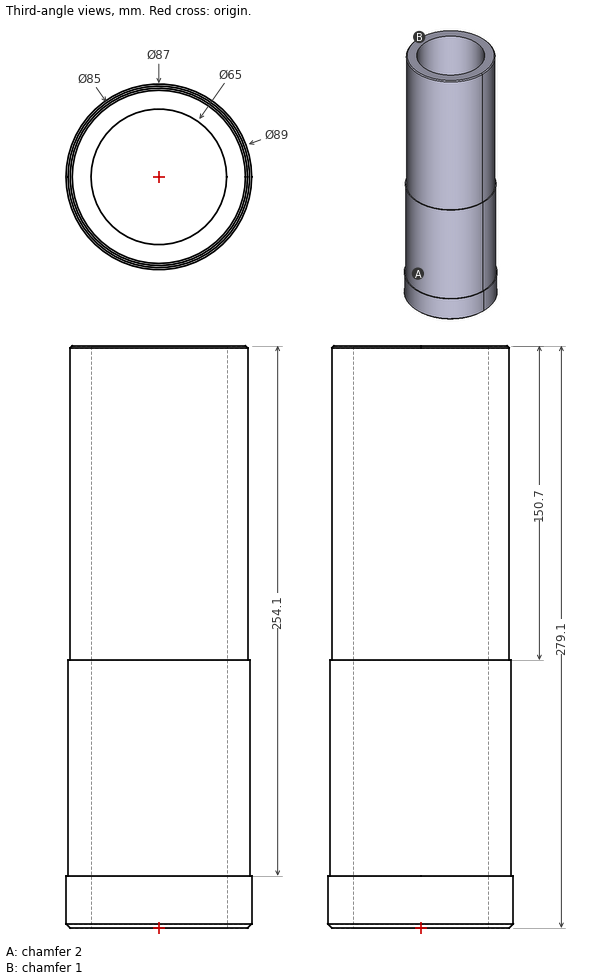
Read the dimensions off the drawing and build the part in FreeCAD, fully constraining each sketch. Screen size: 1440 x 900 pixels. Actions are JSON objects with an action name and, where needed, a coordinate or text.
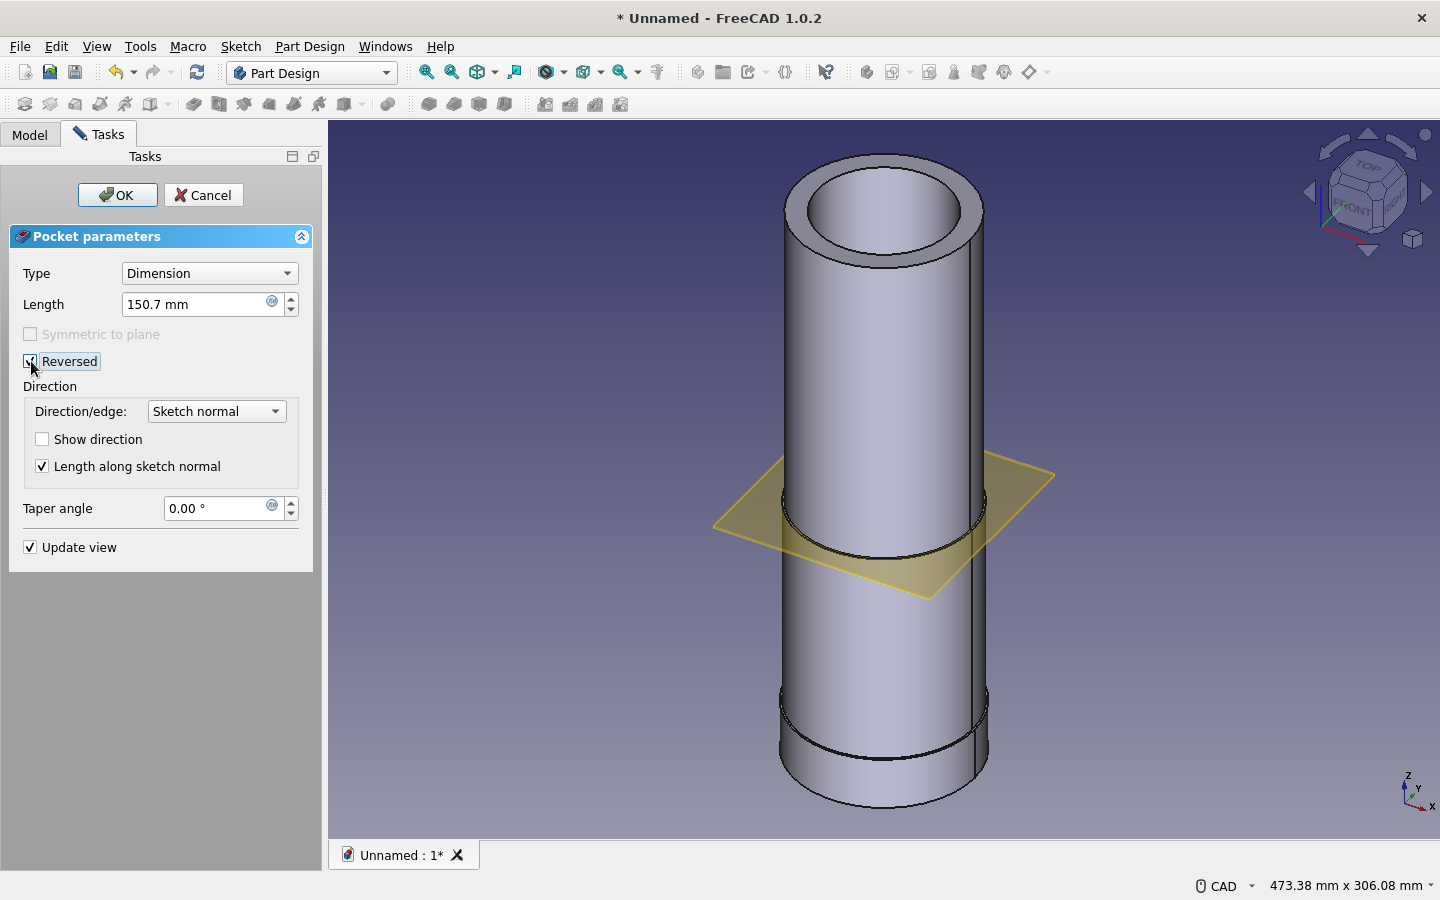
{"action": "left_click", "coordinate": [118, 195]}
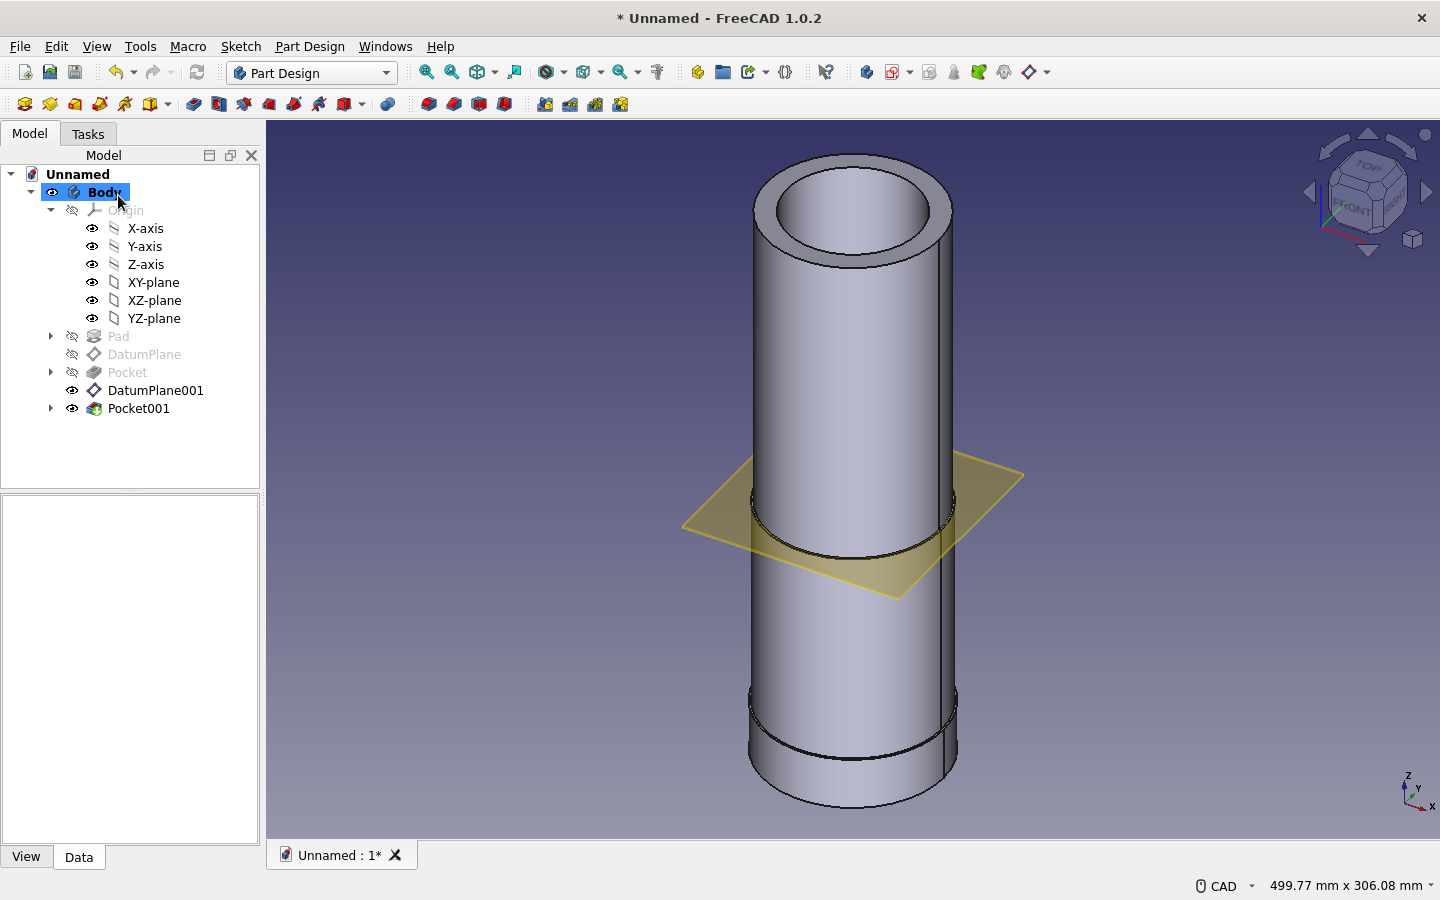
{"action": "left_click", "coordinate": [117, 390]}
{"action": "key", "text": "space"}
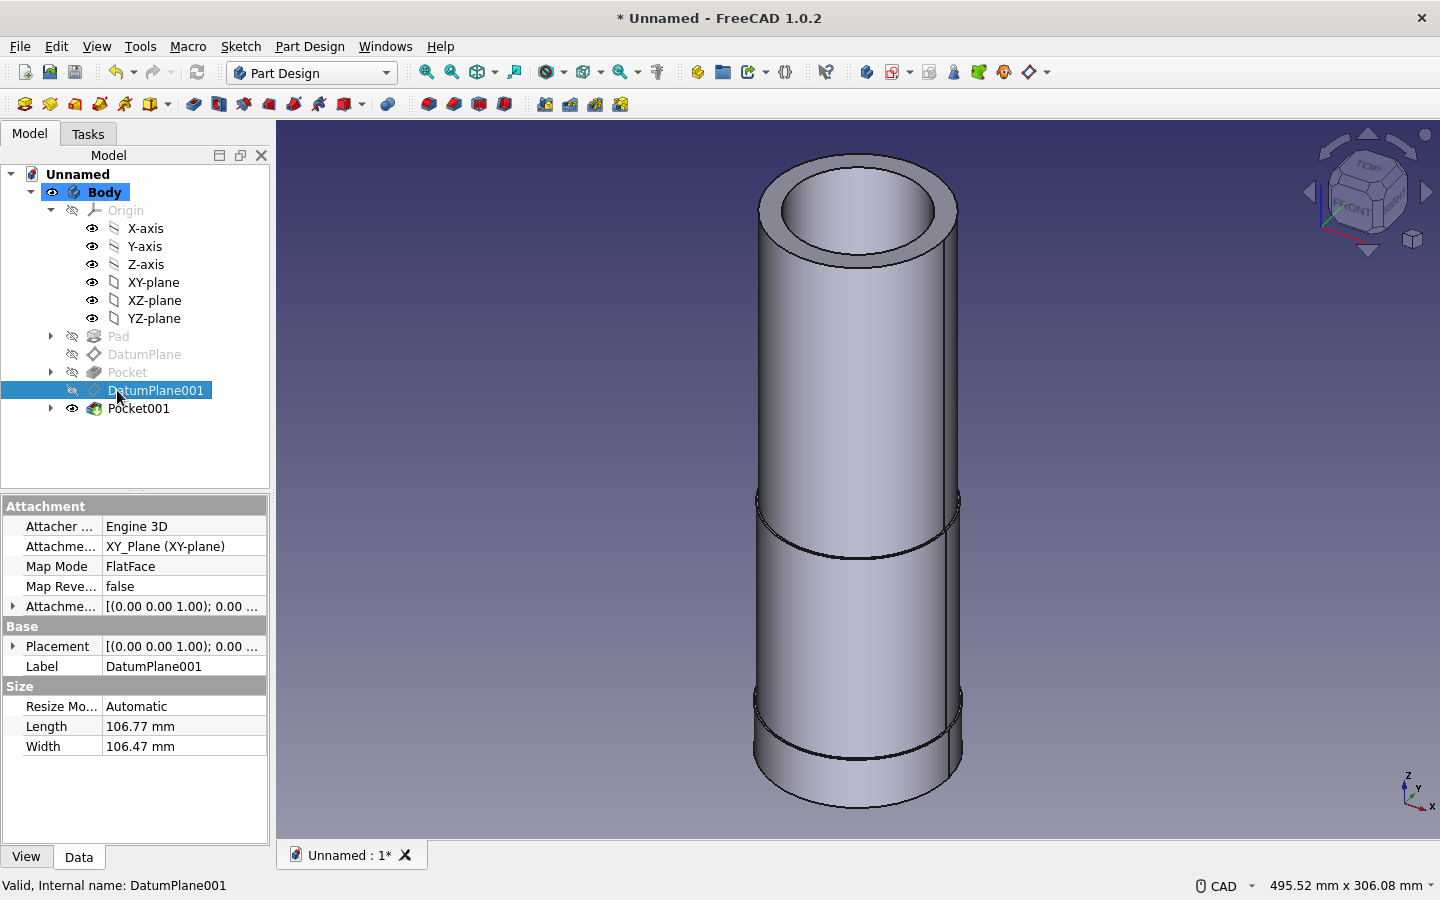
{"action": "key", "text": "0"}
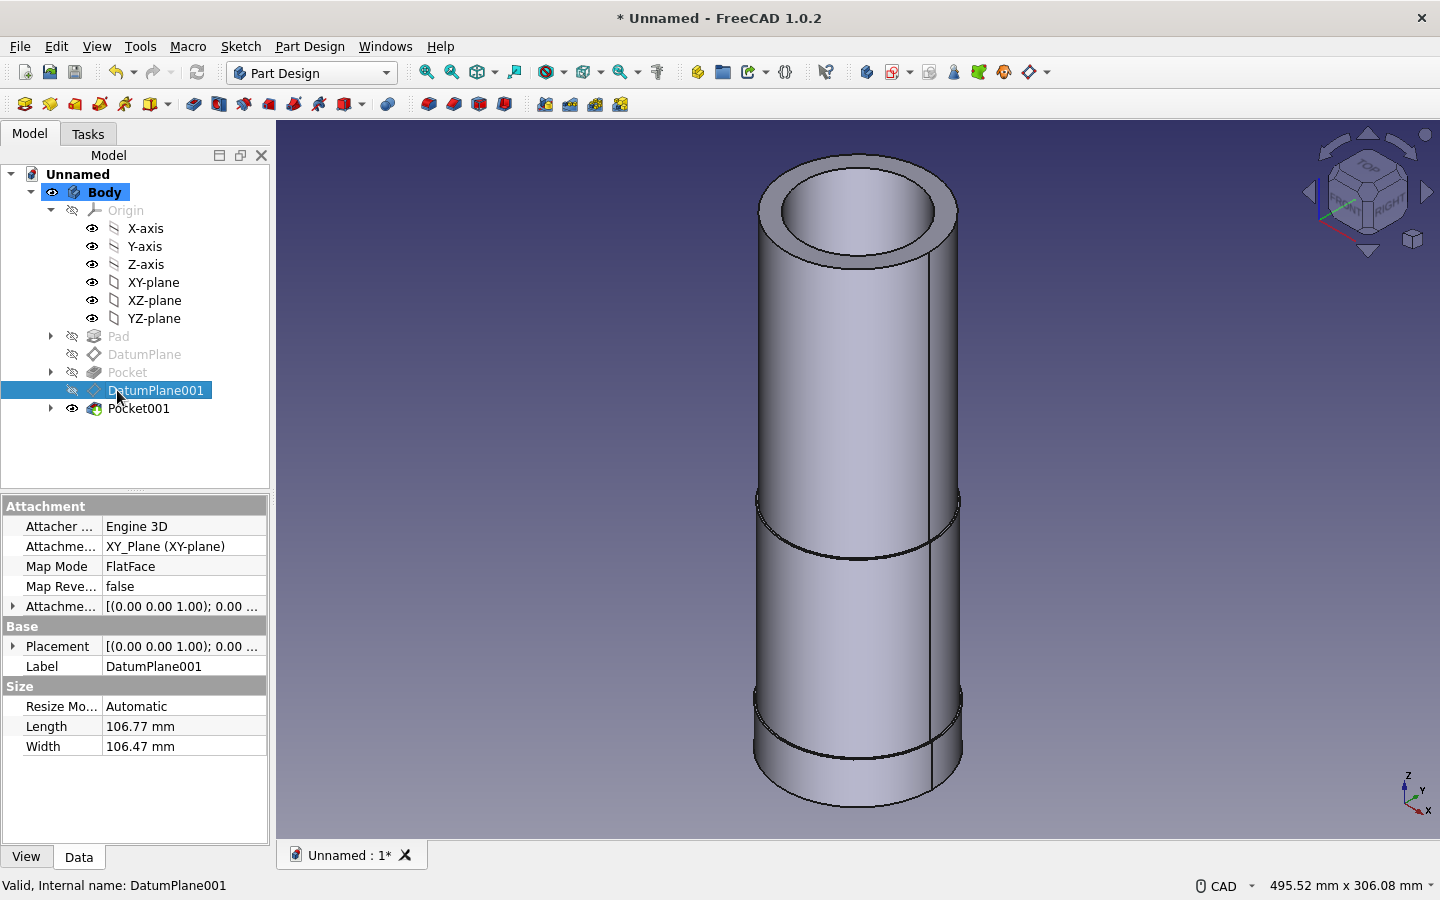
{"action": "key", "text": "2"}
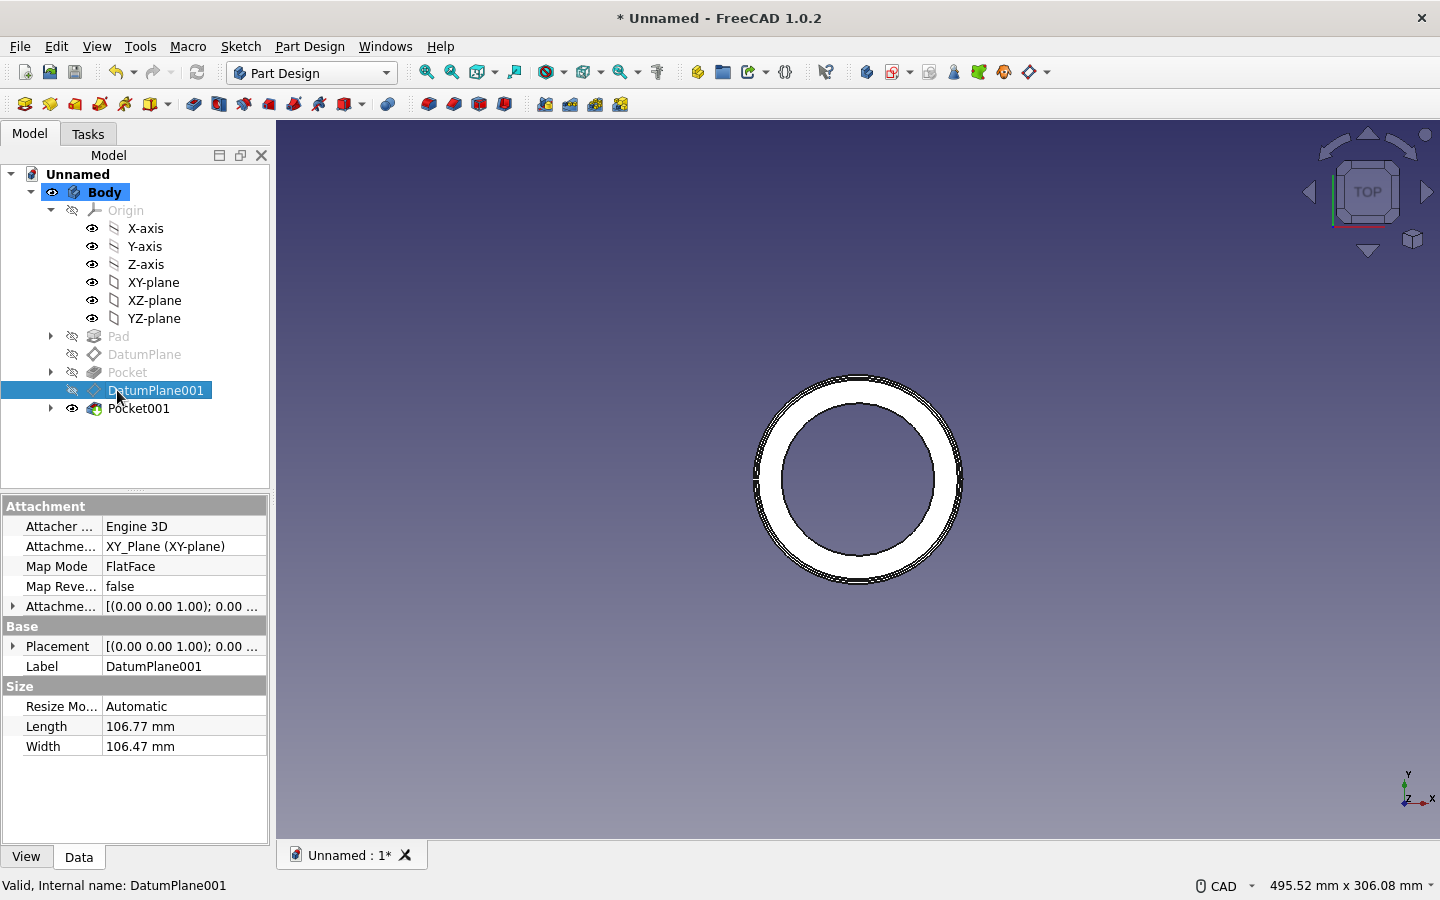
{"action": "left_click", "coordinate": [427, 72]}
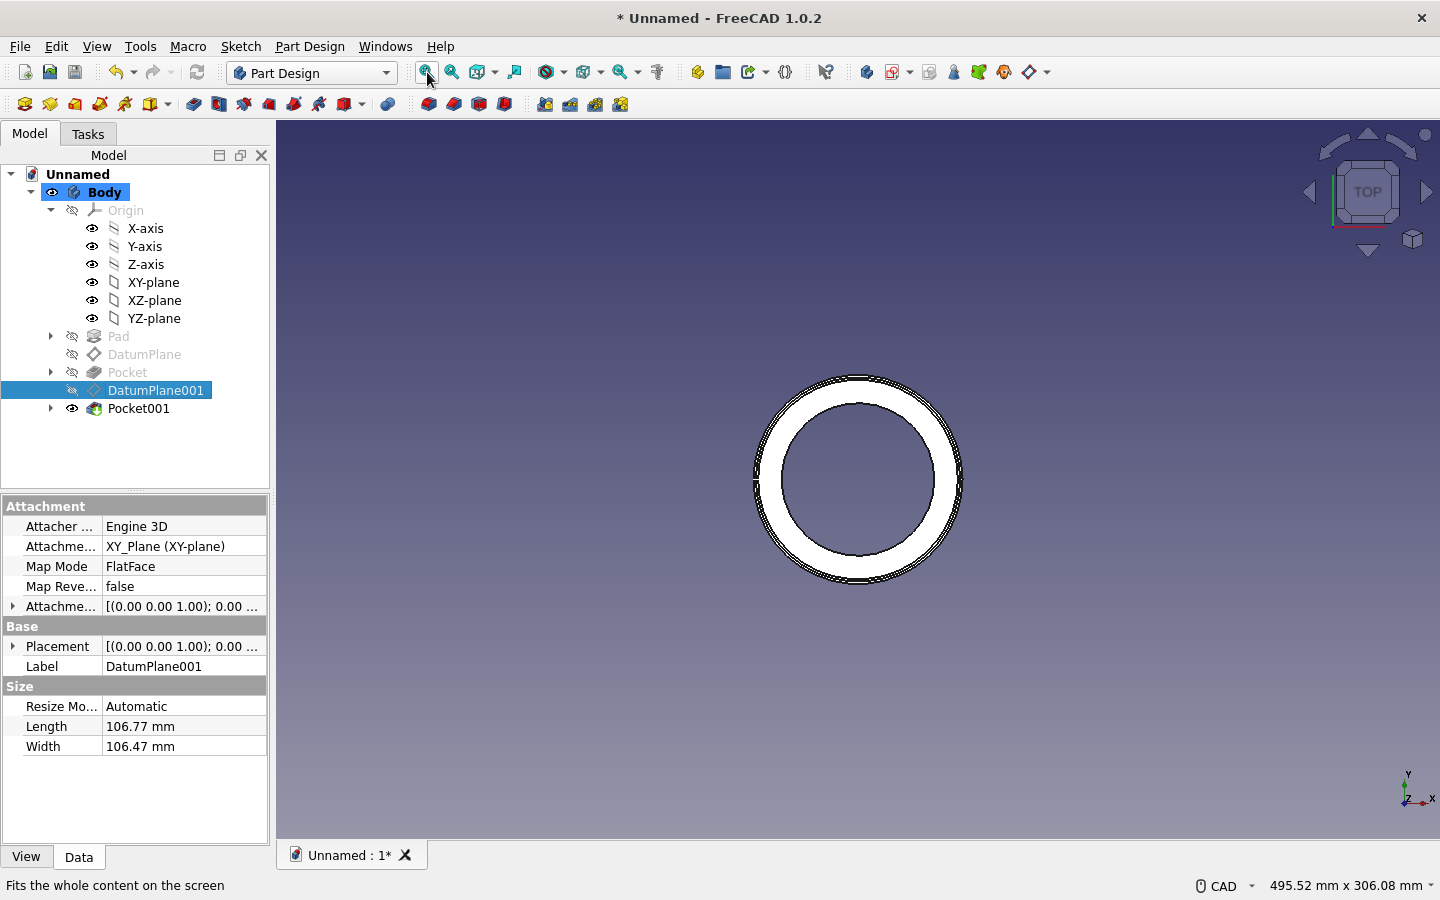
{"action": "key", "text": "1"}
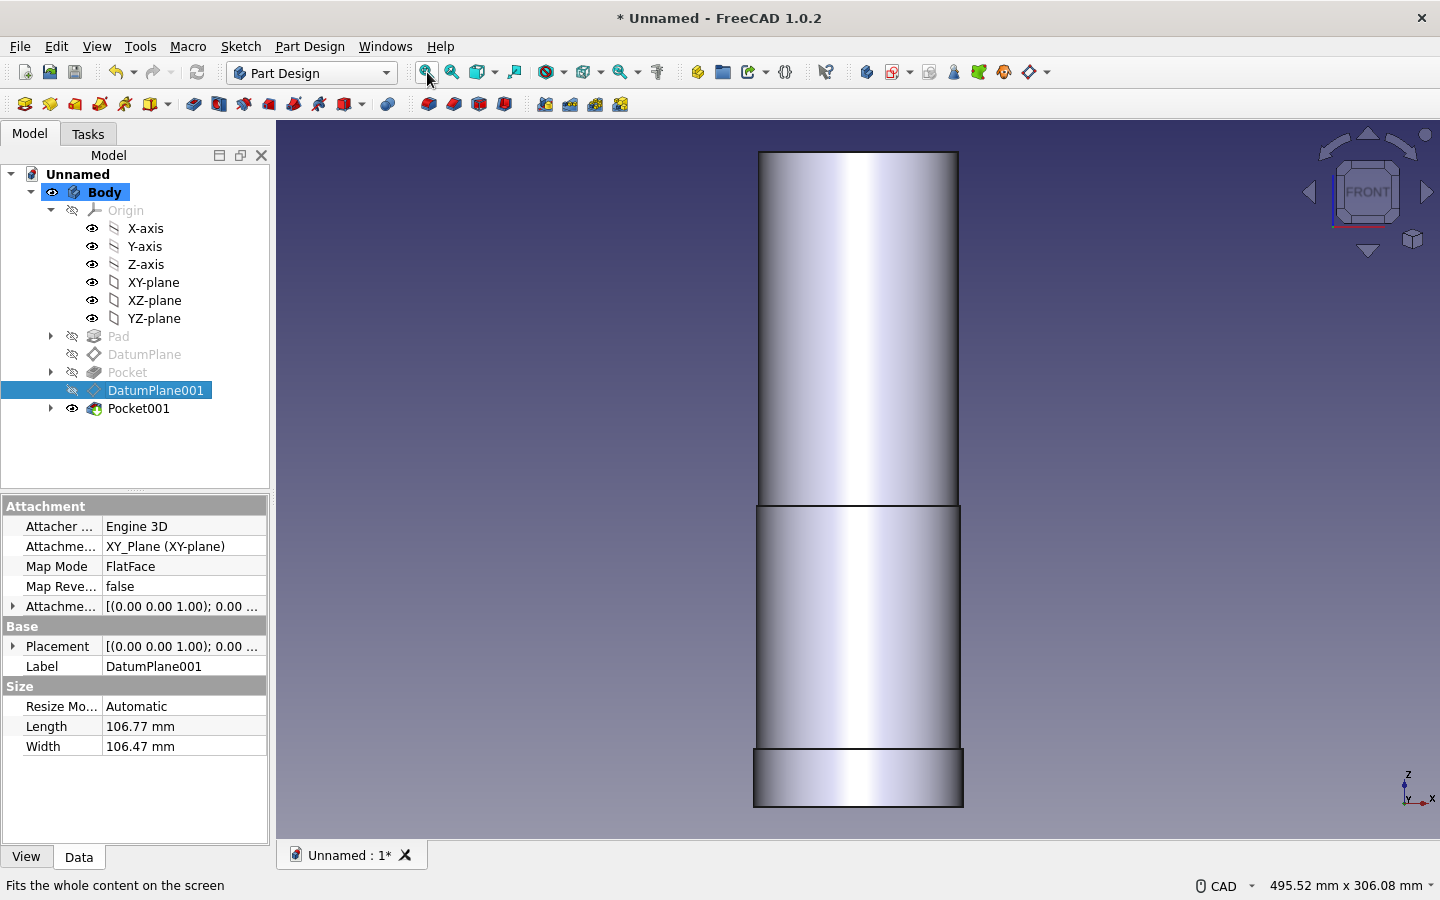
{"action": "left_click", "coordinate": [773, 806]}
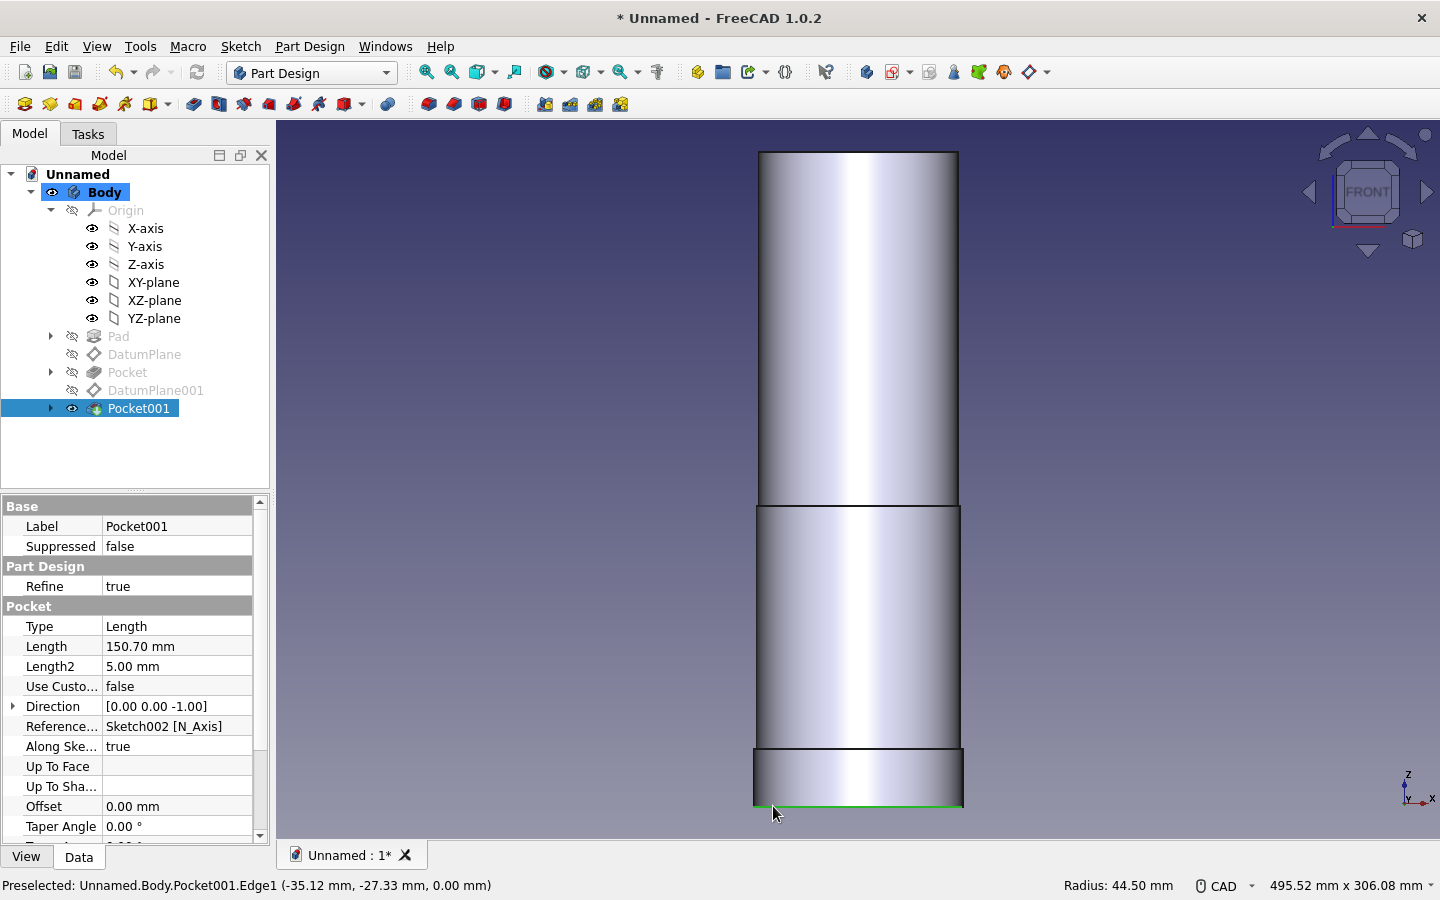
{"action": "left_click", "coordinate": [454, 104]}